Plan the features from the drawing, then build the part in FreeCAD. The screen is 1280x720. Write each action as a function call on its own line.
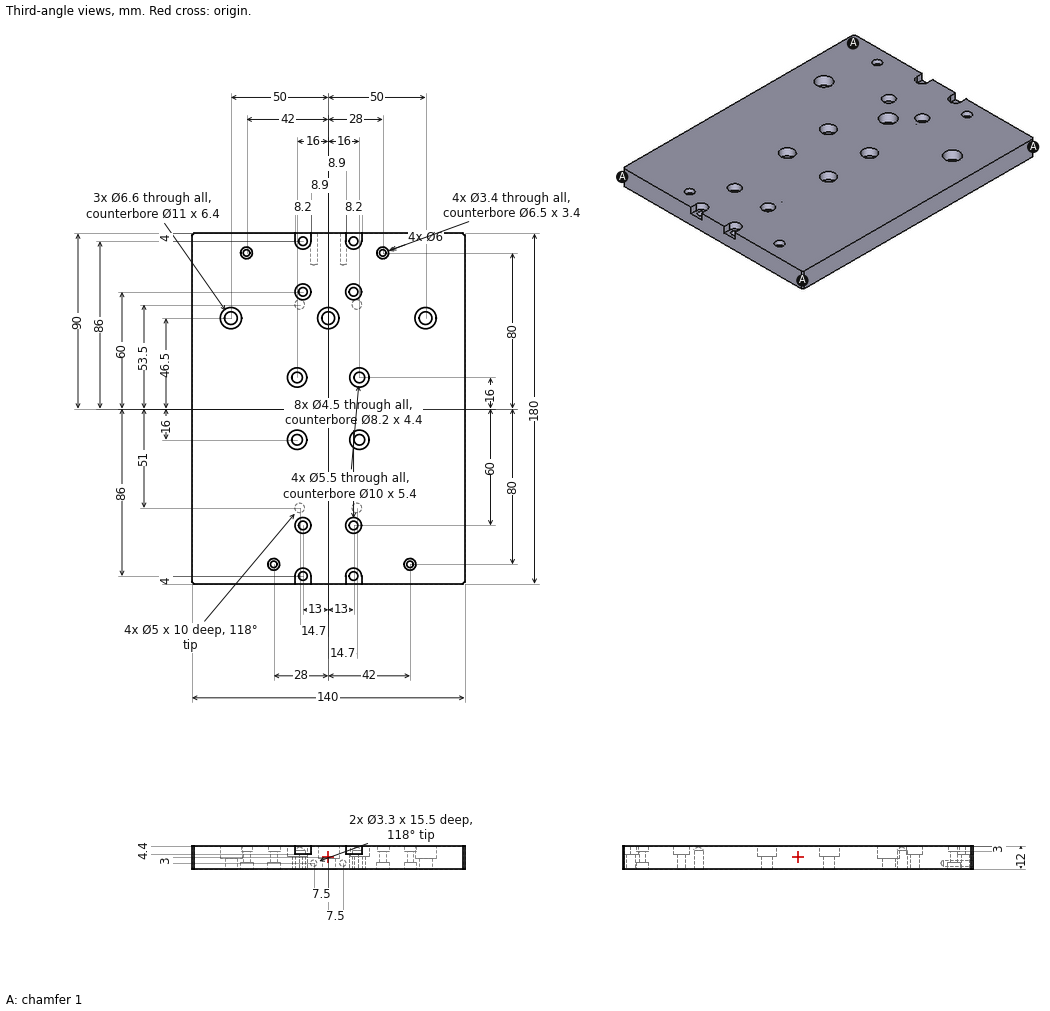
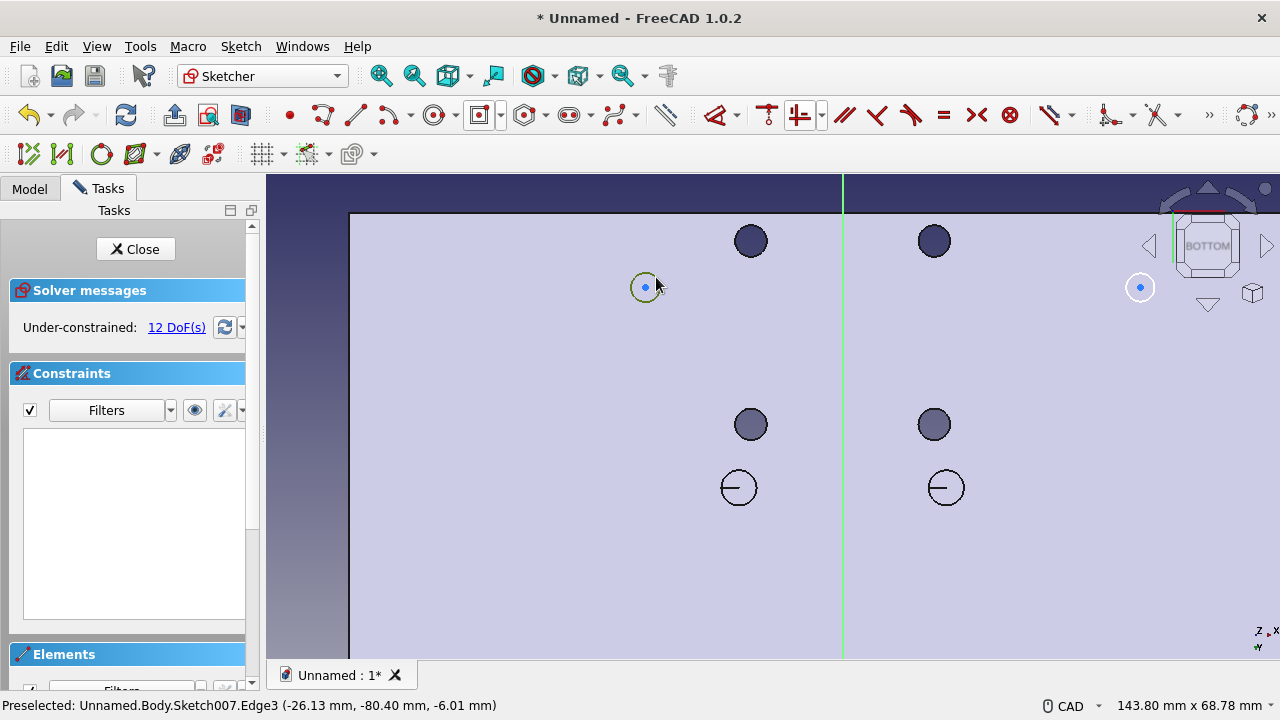
scroll(659, 275, down, 7)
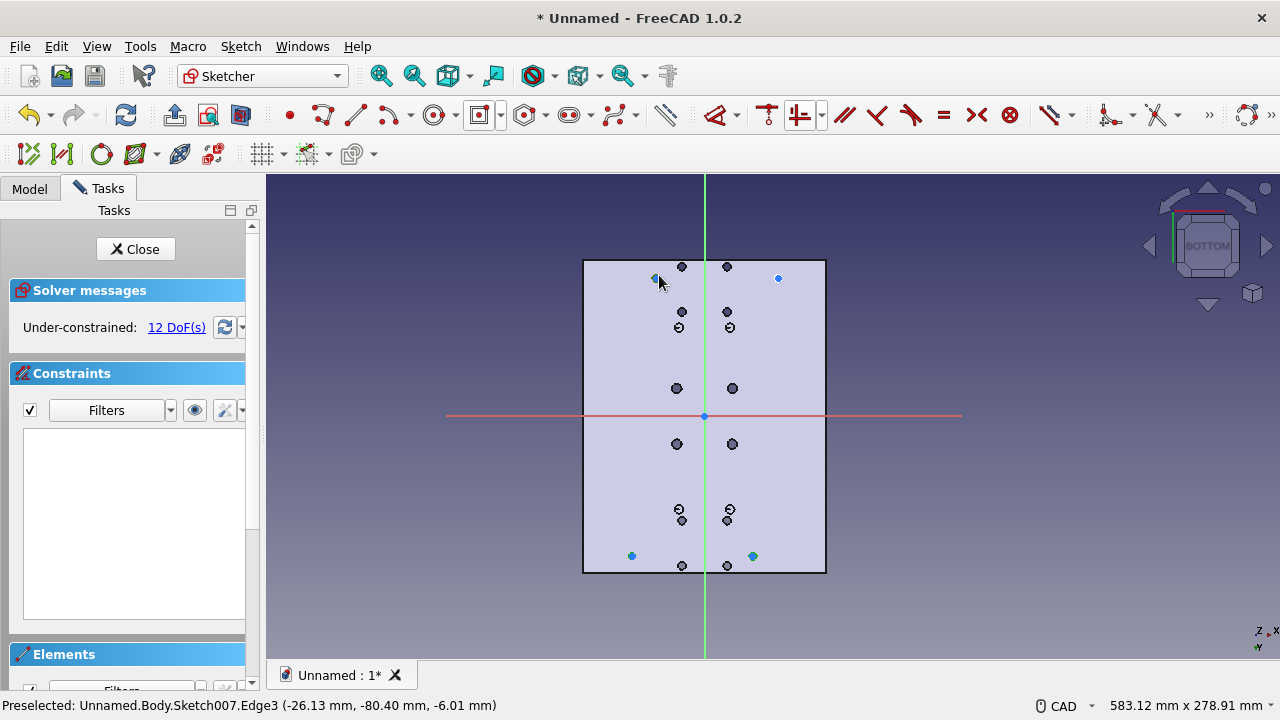
scroll(780, 276, up, 7)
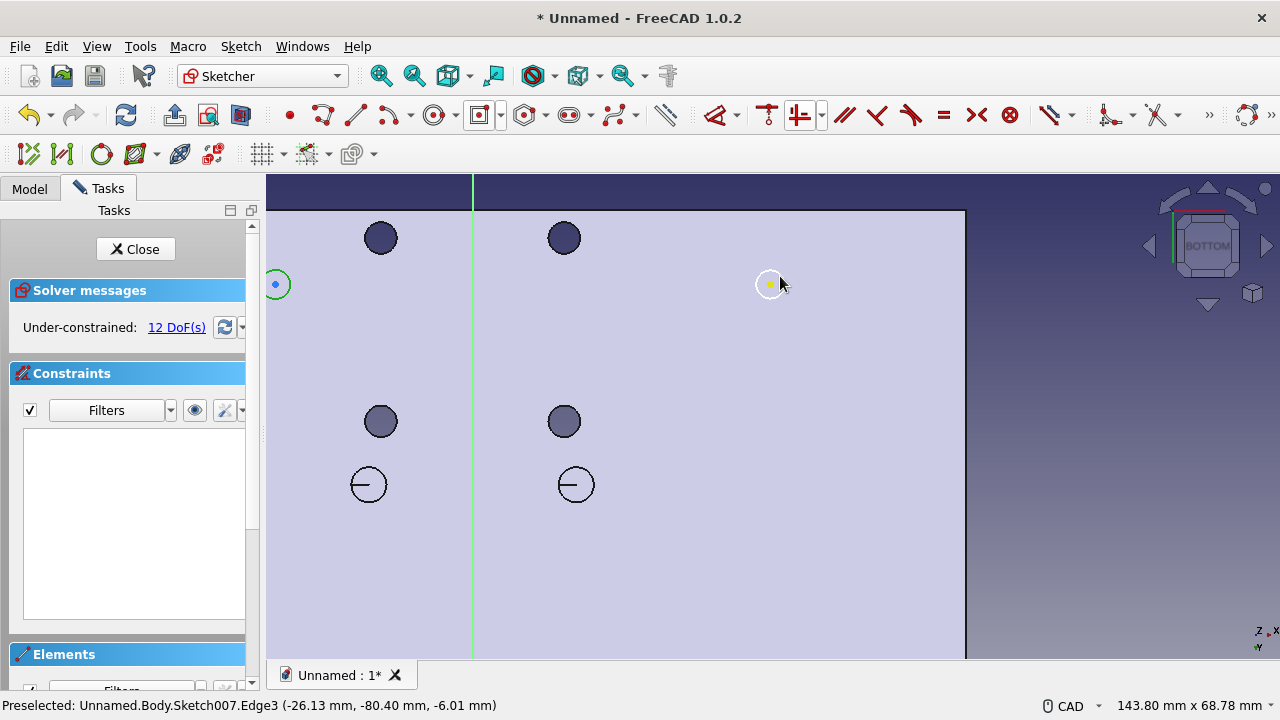
click(780, 274)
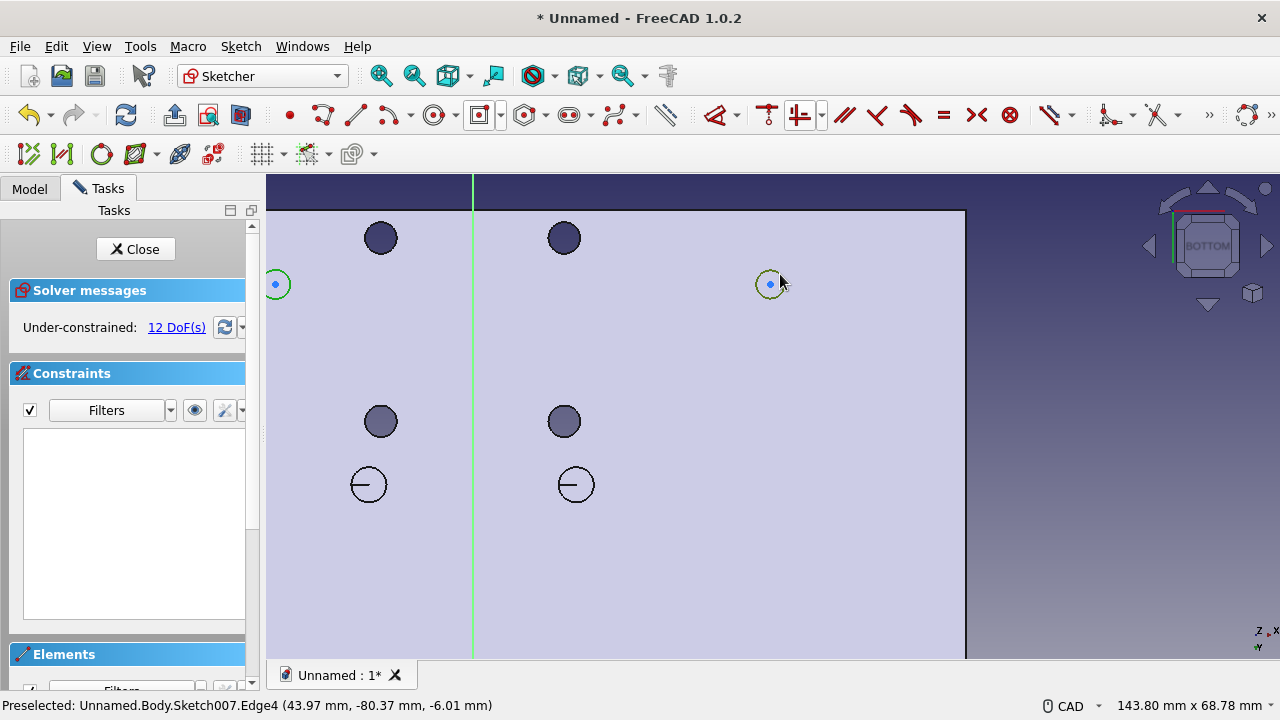
click(944, 116)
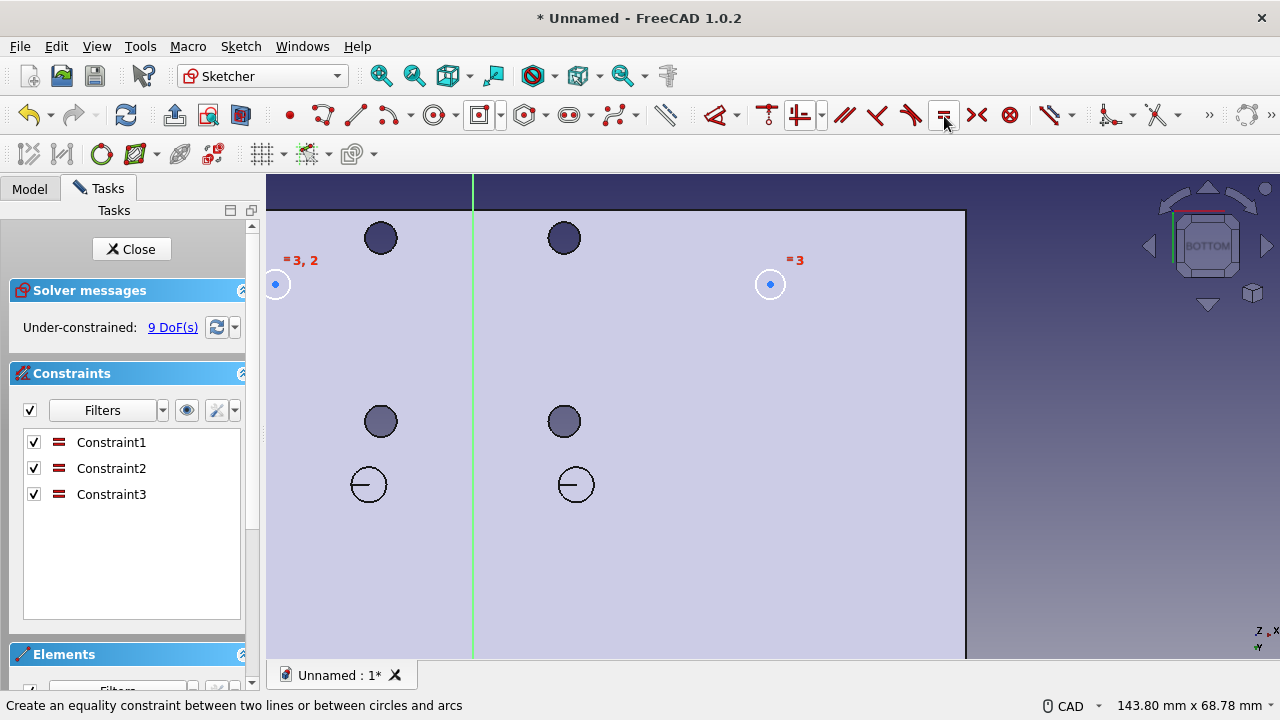
click(714, 116)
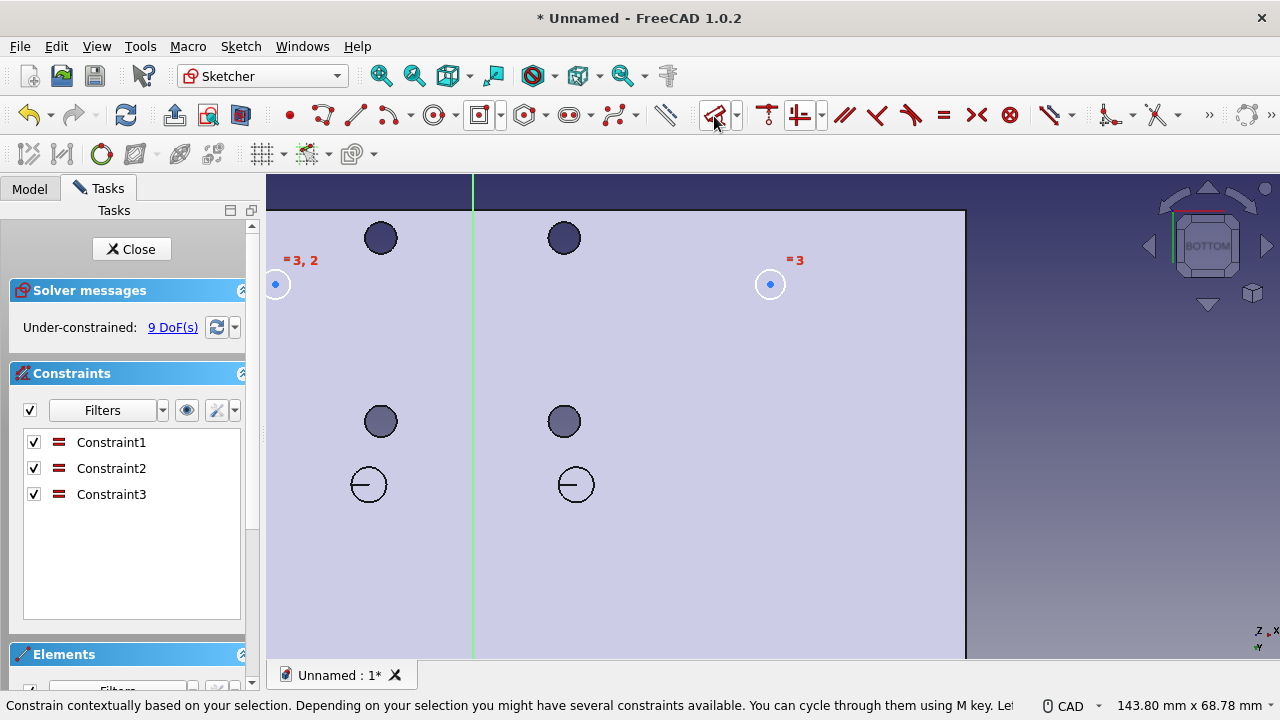
scroll(780, 276, down, 7)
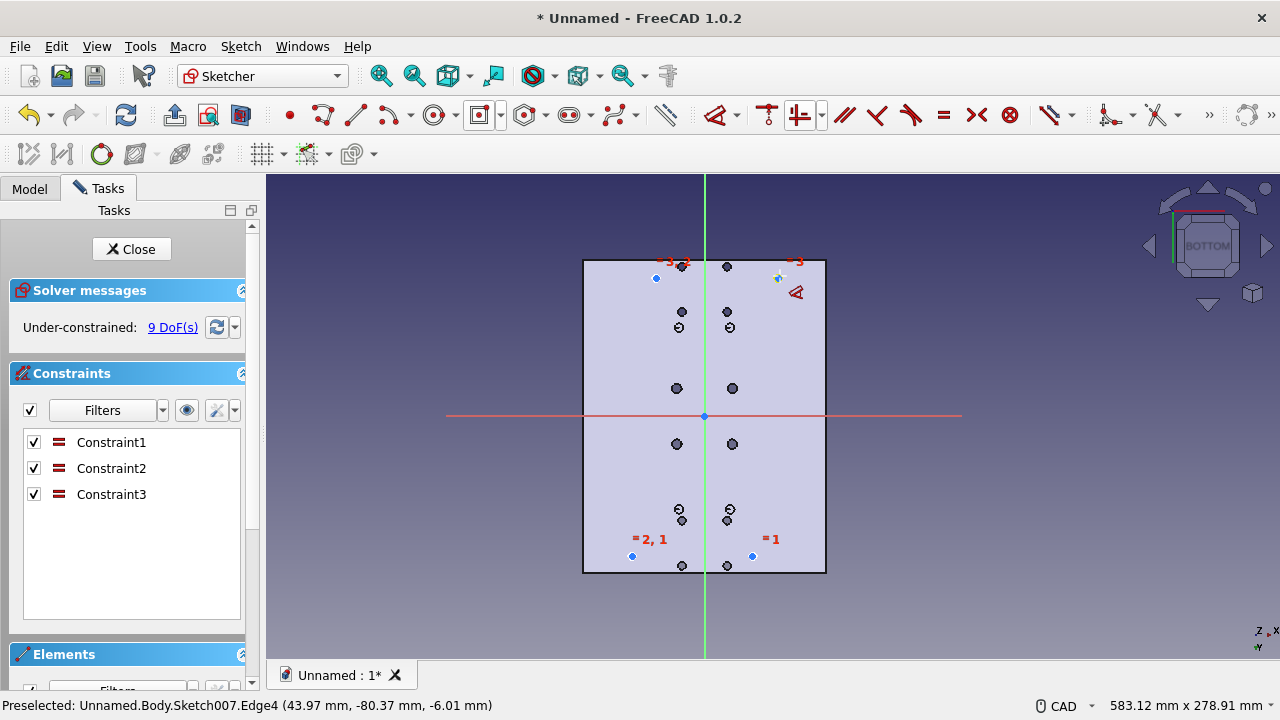
scroll(756, 554, up, 10)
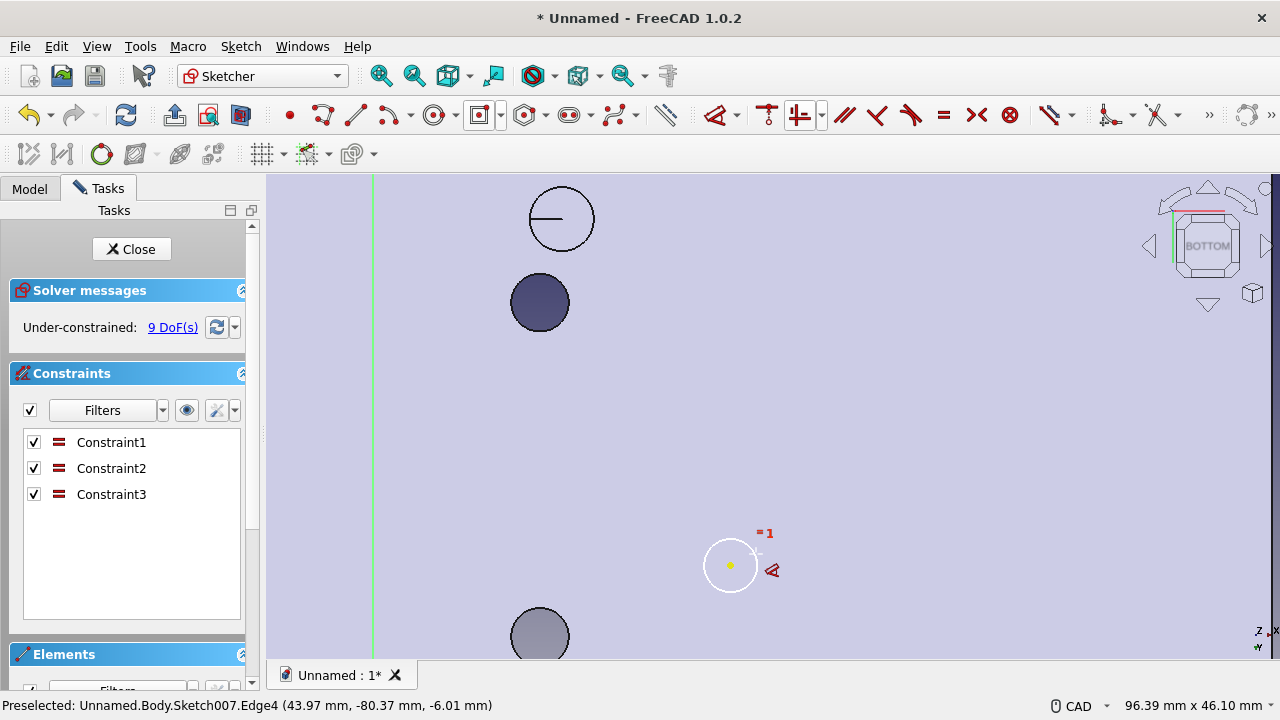
click(749, 547)
click(771, 524)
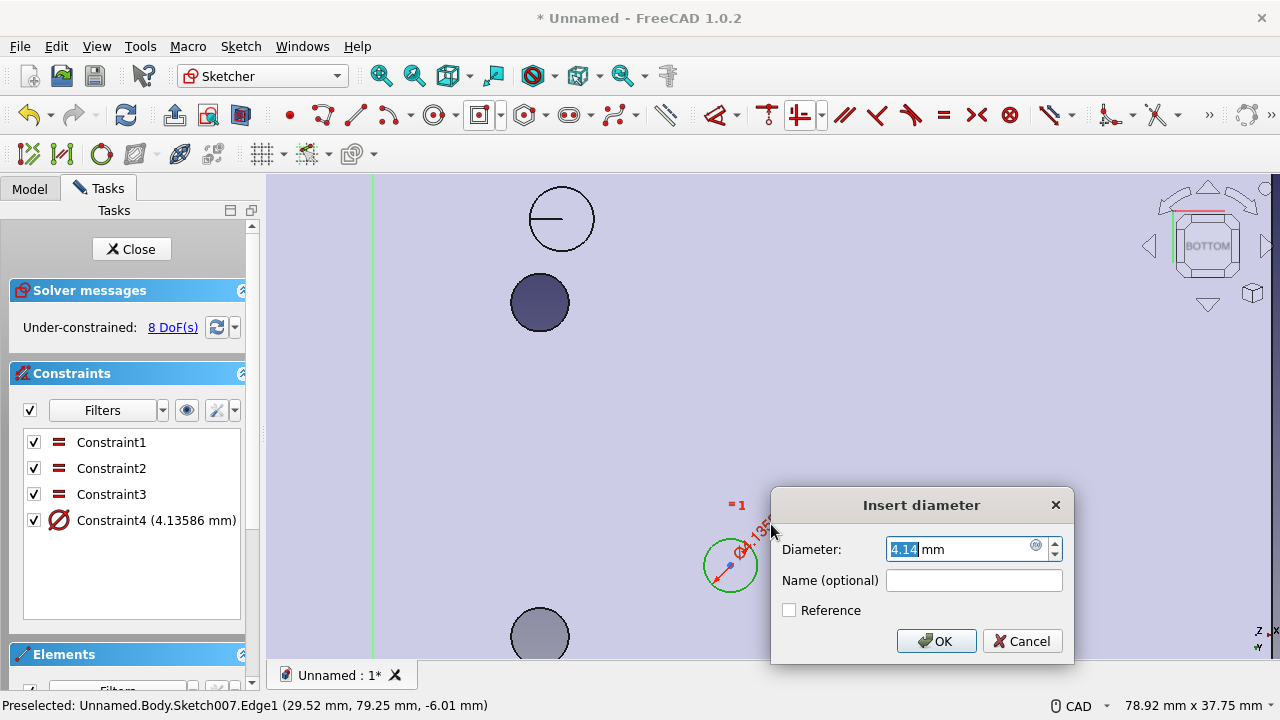
text(3.4)
key(Return)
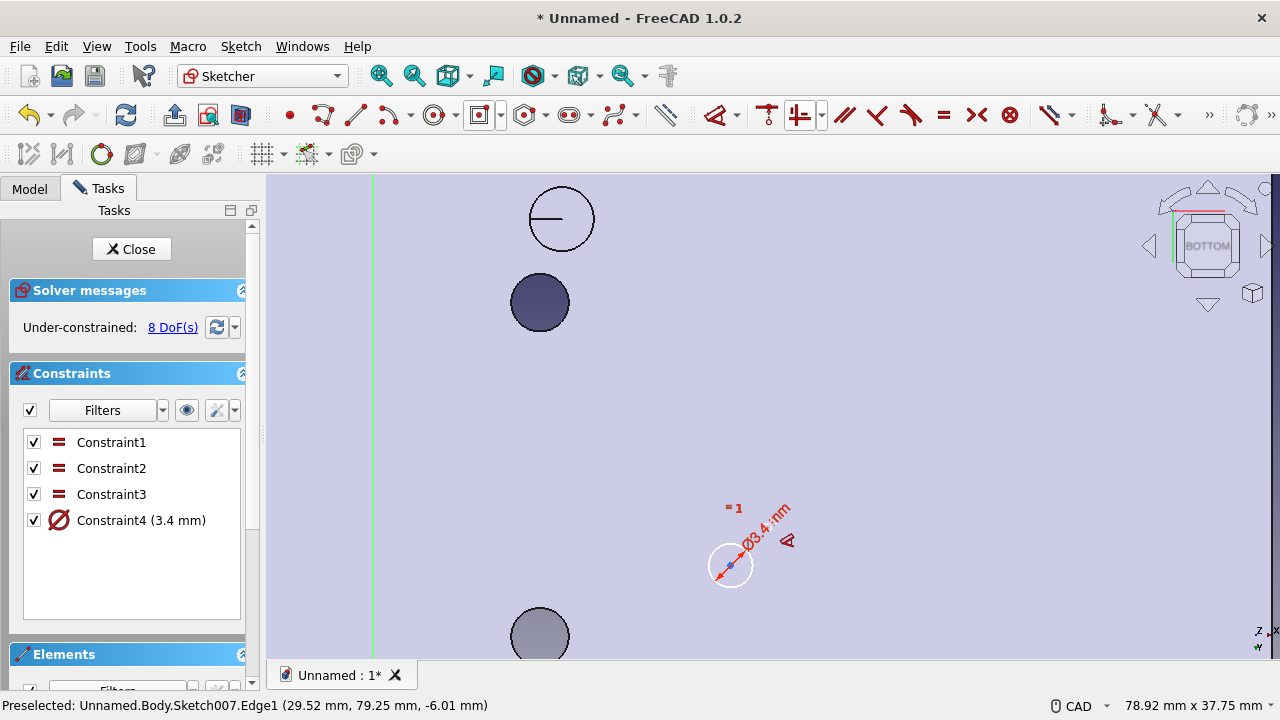
scroll(756, 555, down, 10)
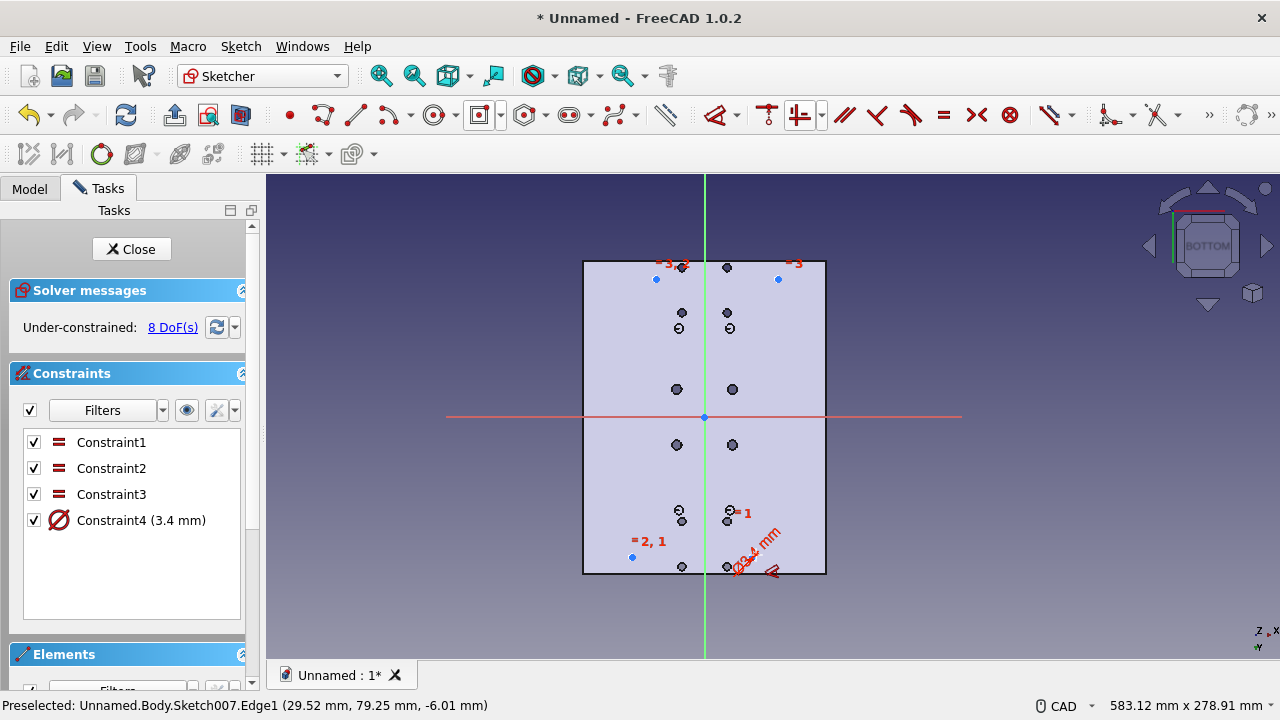
click(753, 557)
click(729, 591)